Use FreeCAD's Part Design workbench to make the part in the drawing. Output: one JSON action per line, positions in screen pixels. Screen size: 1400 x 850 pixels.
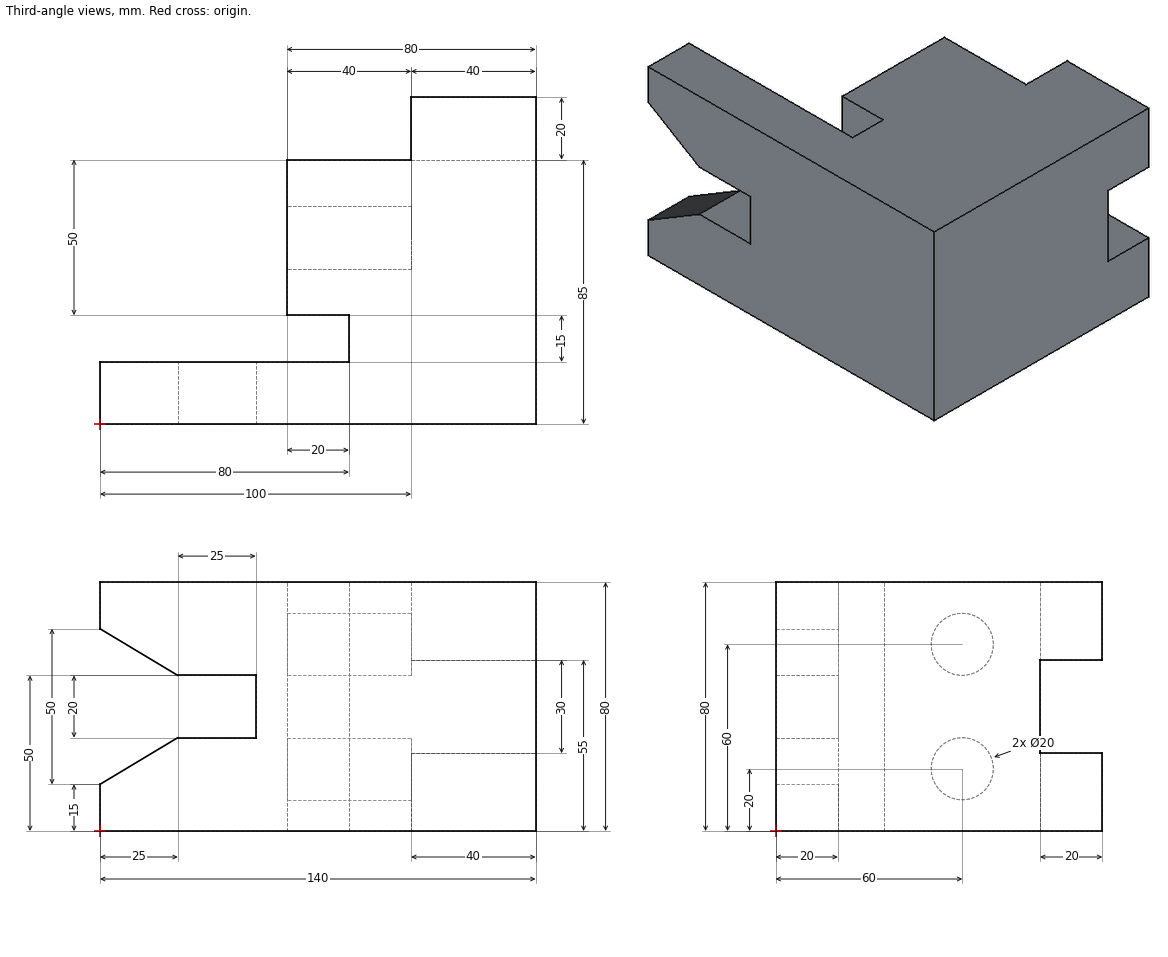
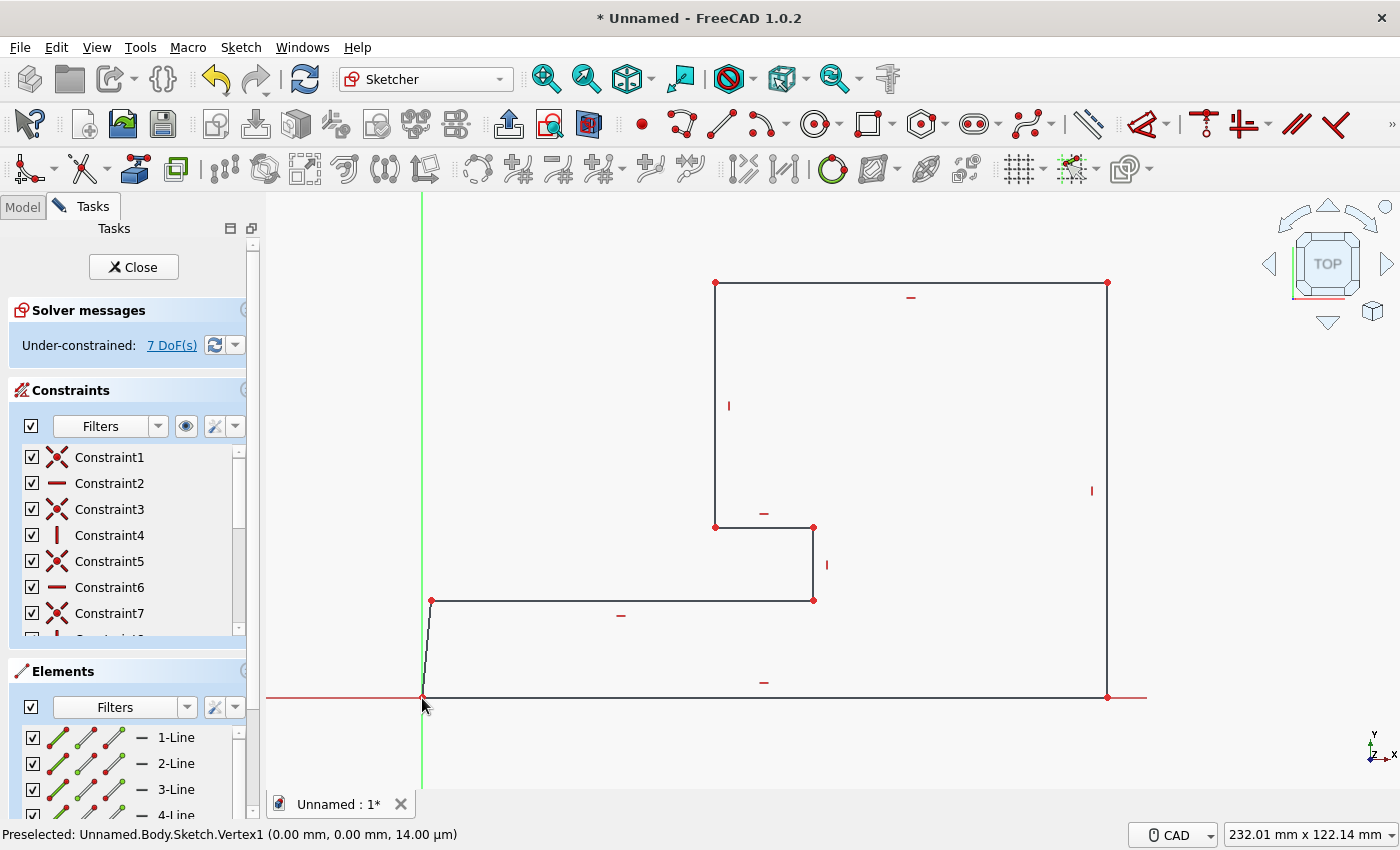
{"action": "left_click", "coordinate": [425, 669]}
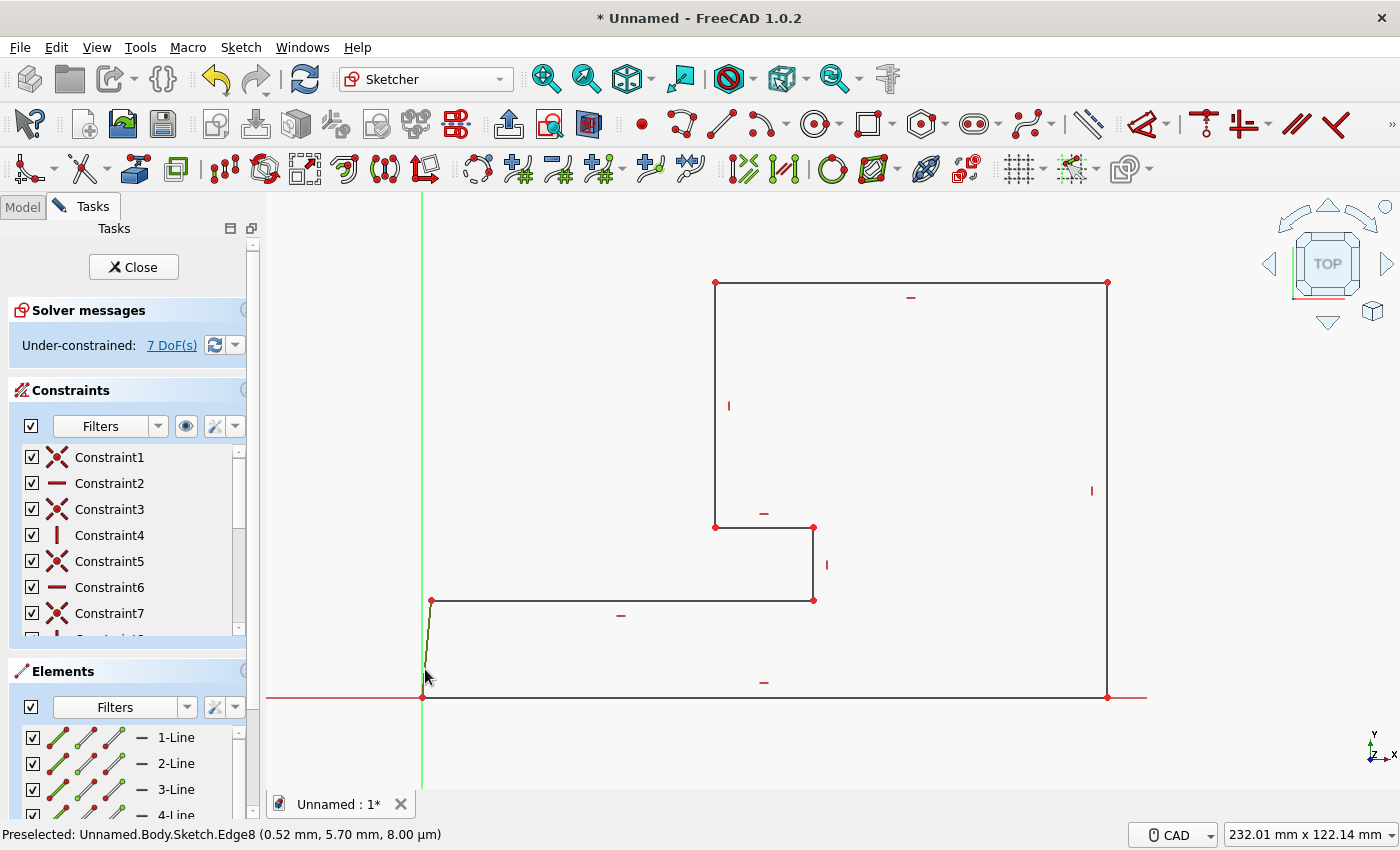
{"action": "key", "text": "v"}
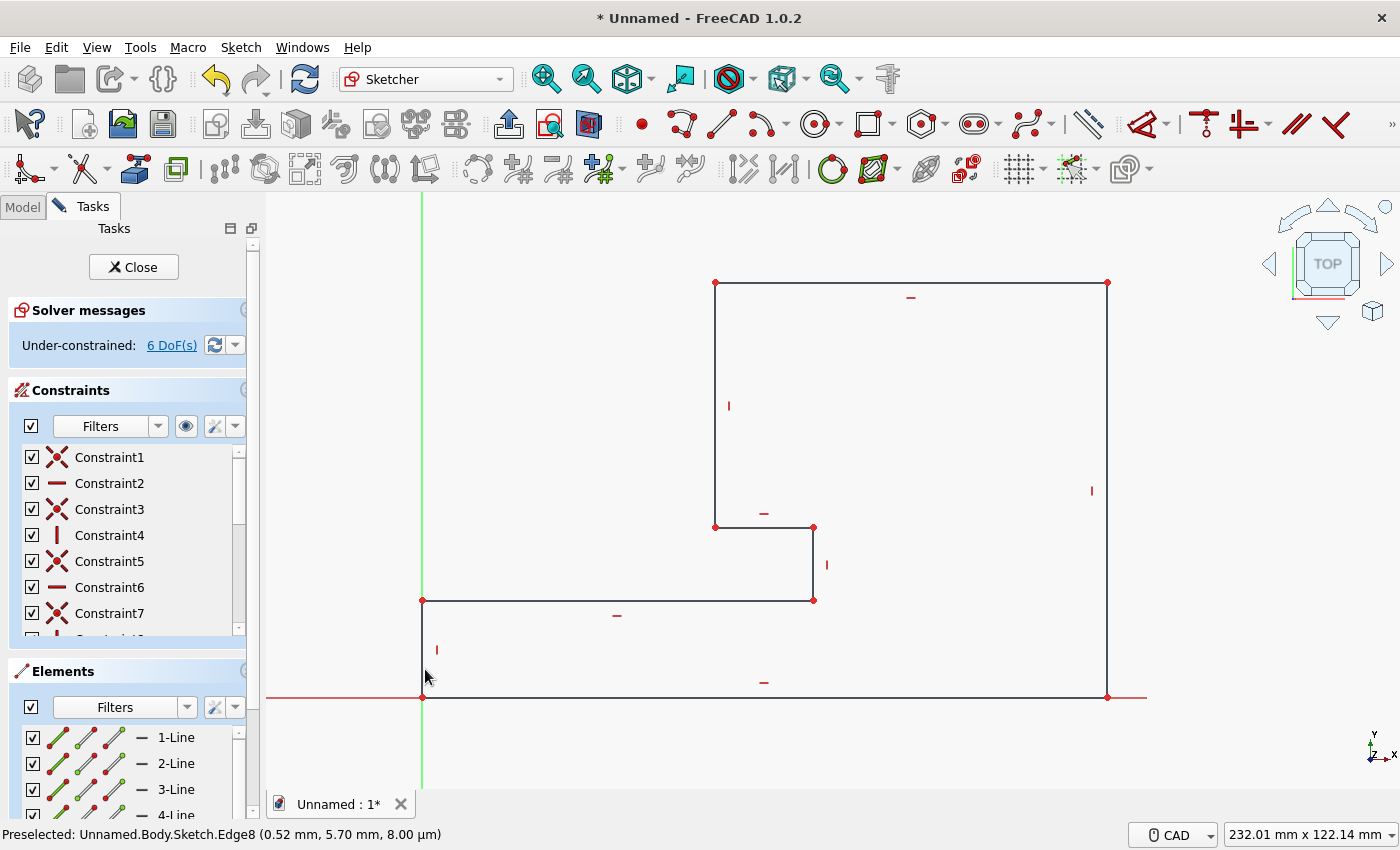
{"action": "left_click", "coordinate": [1142, 124]}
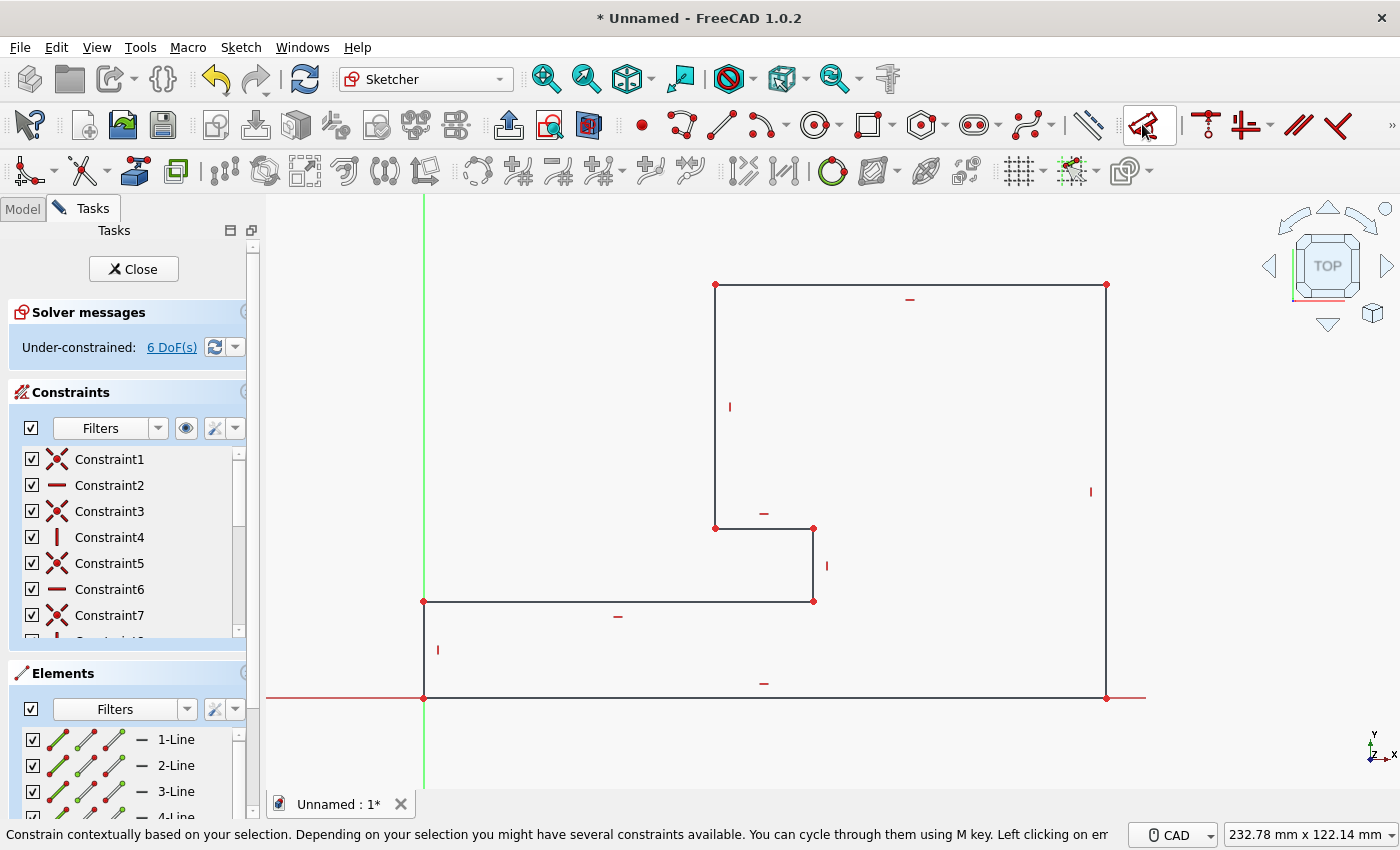
{"action": "left_click", "coordinate": [1106, 574]}
{"action": "left_click", "coordinate": [1140, 491]}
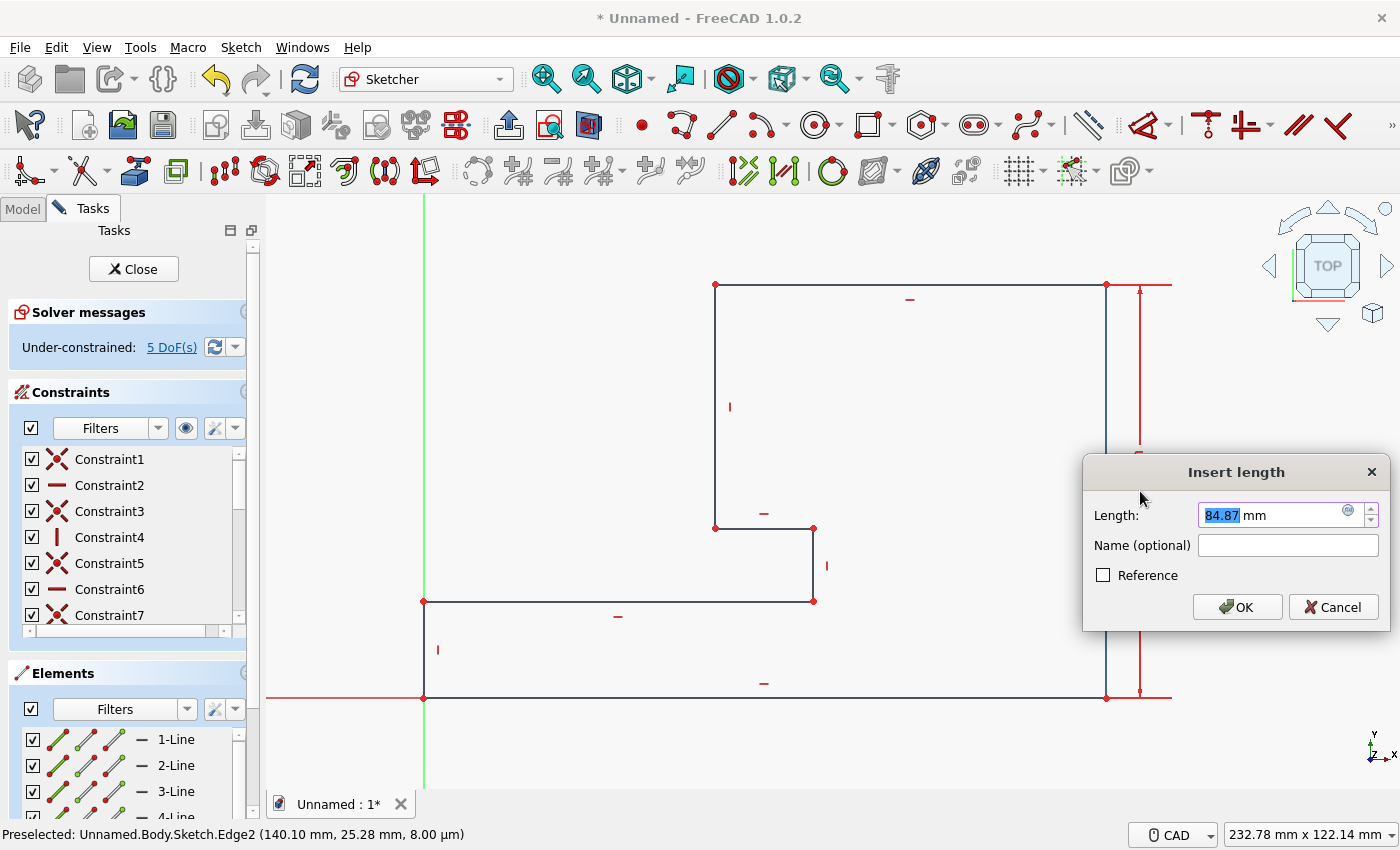
{"action": "type", "text": "85"}
{"action": "key", "text": "Return"}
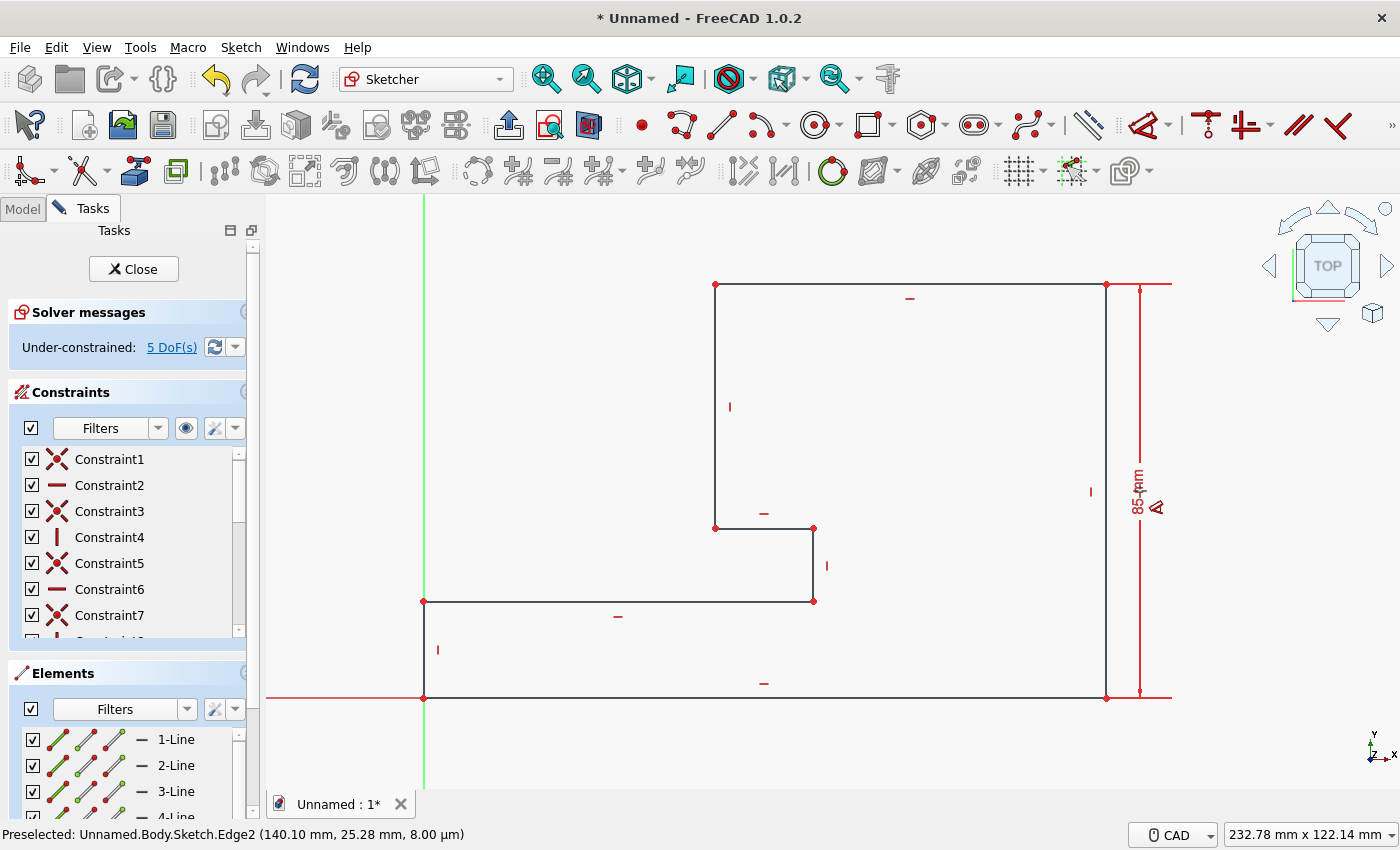
{"action": "left_click", "coordinate": [989, 284]}
{"action": "left_click", "coordinate": [911, 250]}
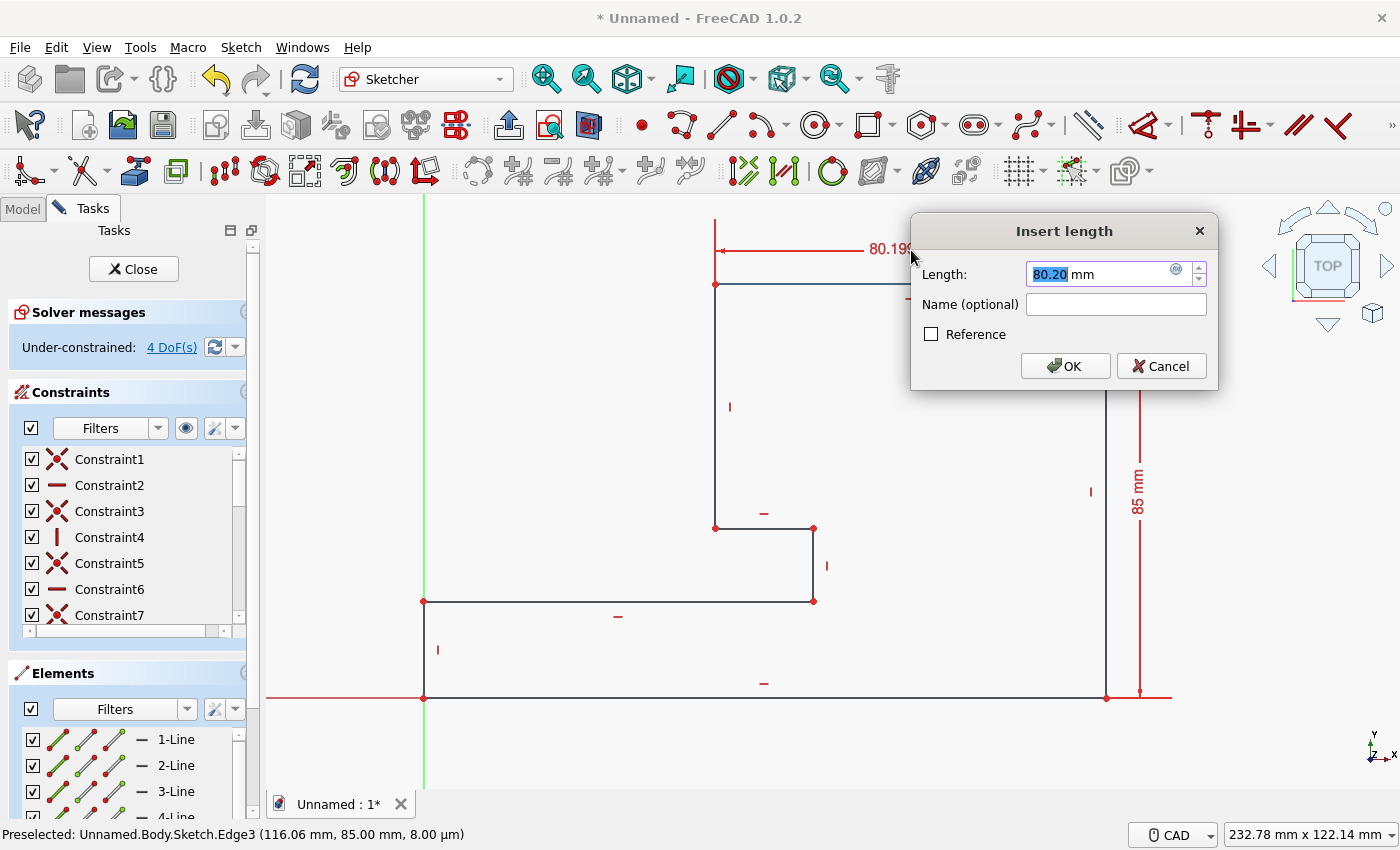
{"action": "type", "text": "80"}
{"action": "key", "text": "Return"}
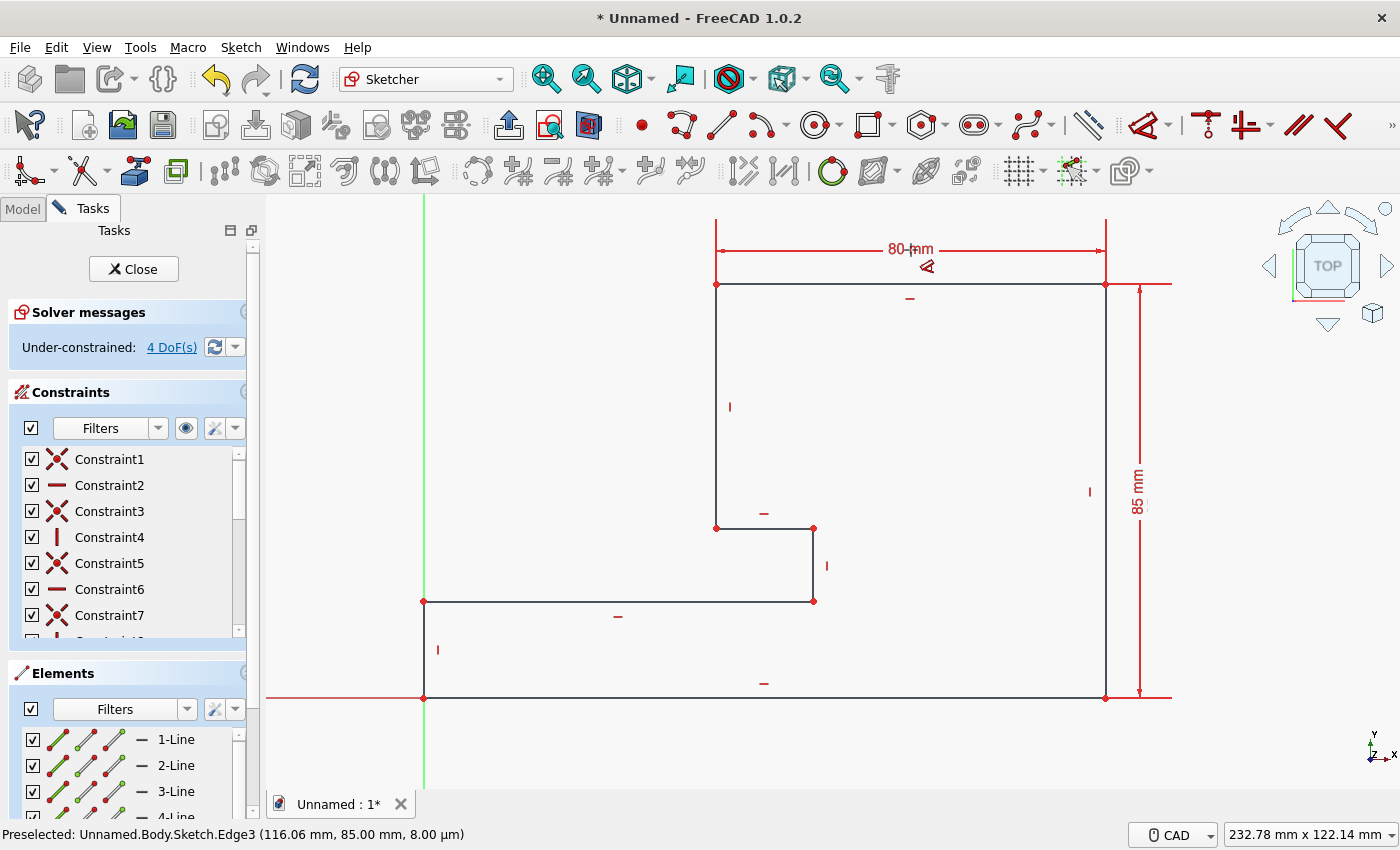
{"action": "left_click", "coordinate": [716, 358]}
{"action": "left_click", "coordinate": [682, 406]}